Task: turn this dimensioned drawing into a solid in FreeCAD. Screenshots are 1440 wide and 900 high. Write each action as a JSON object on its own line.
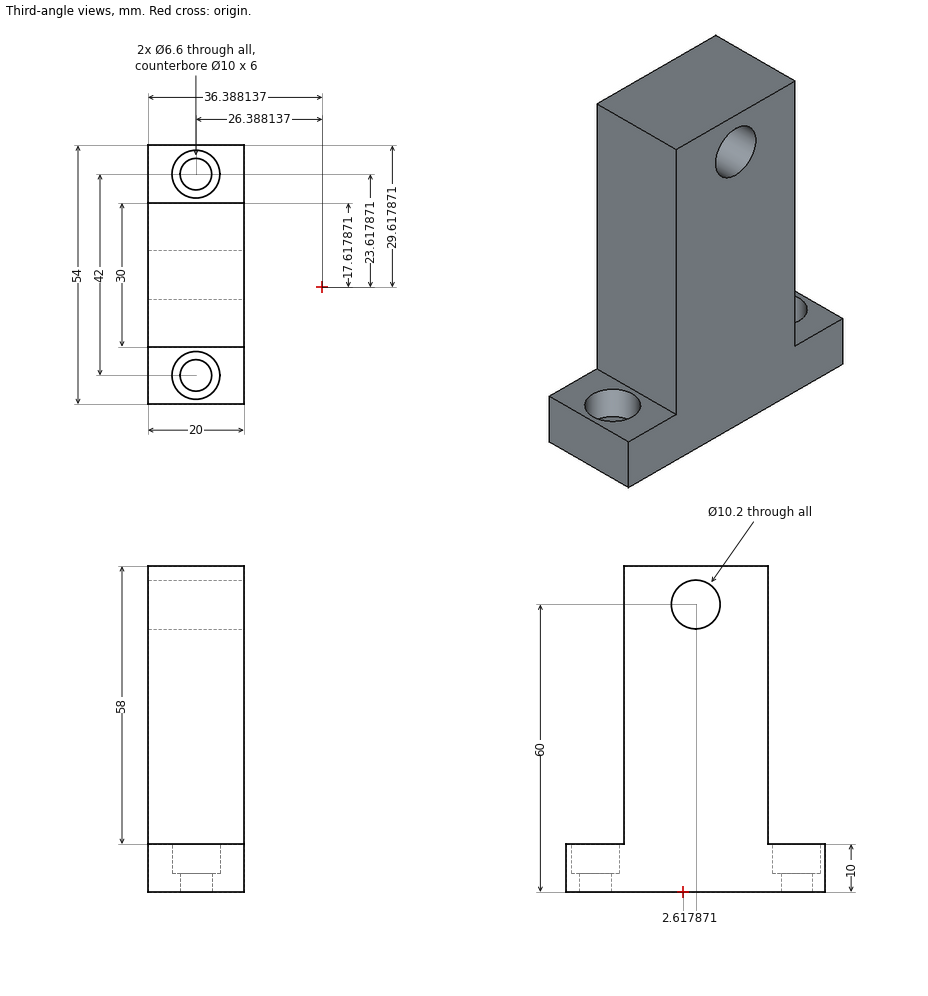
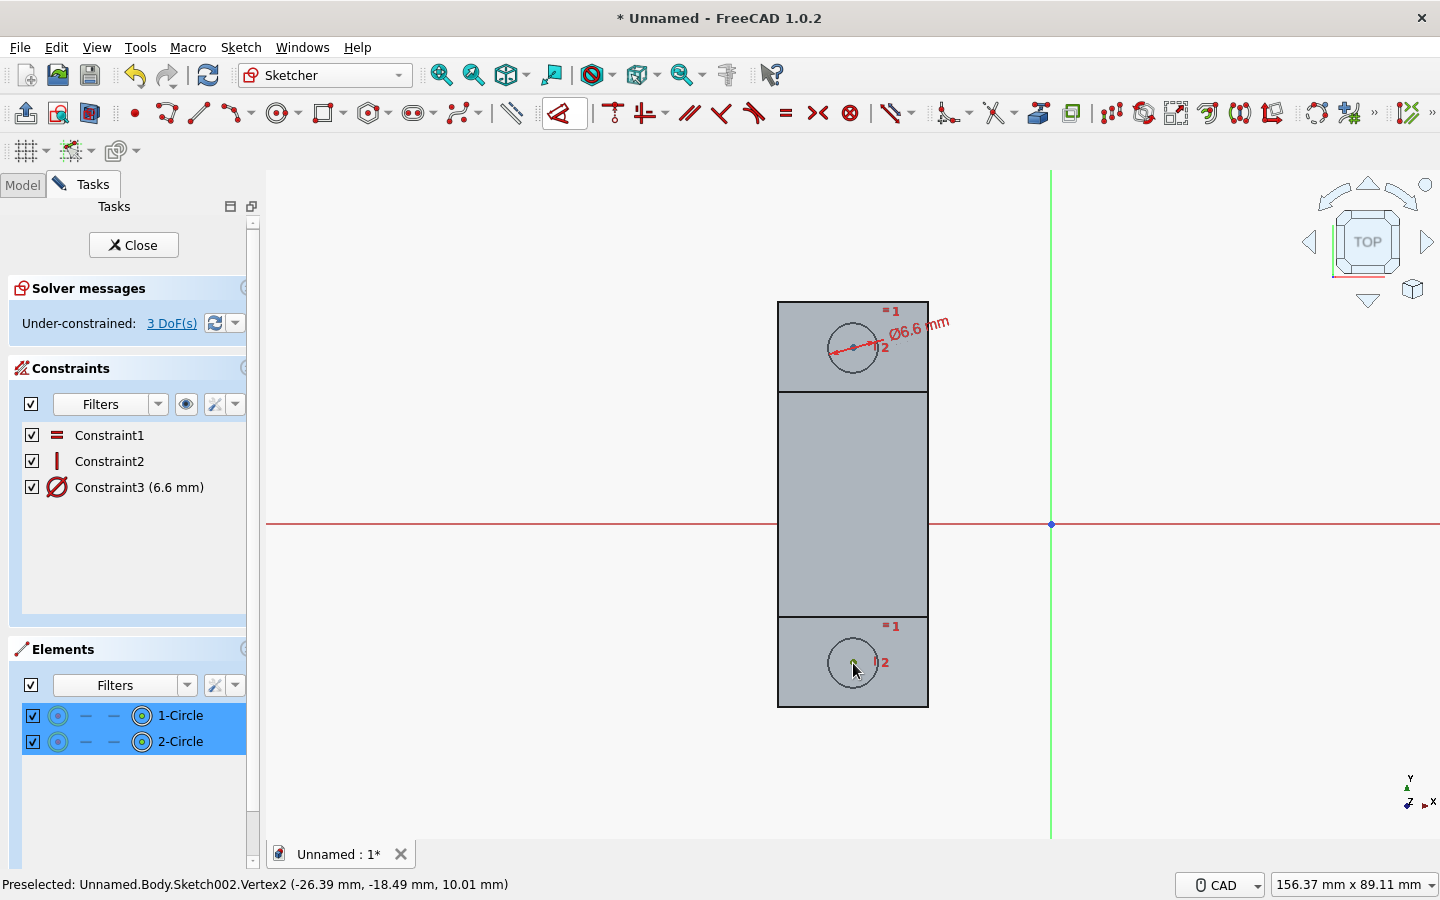
{"action": "key", "text": "i"}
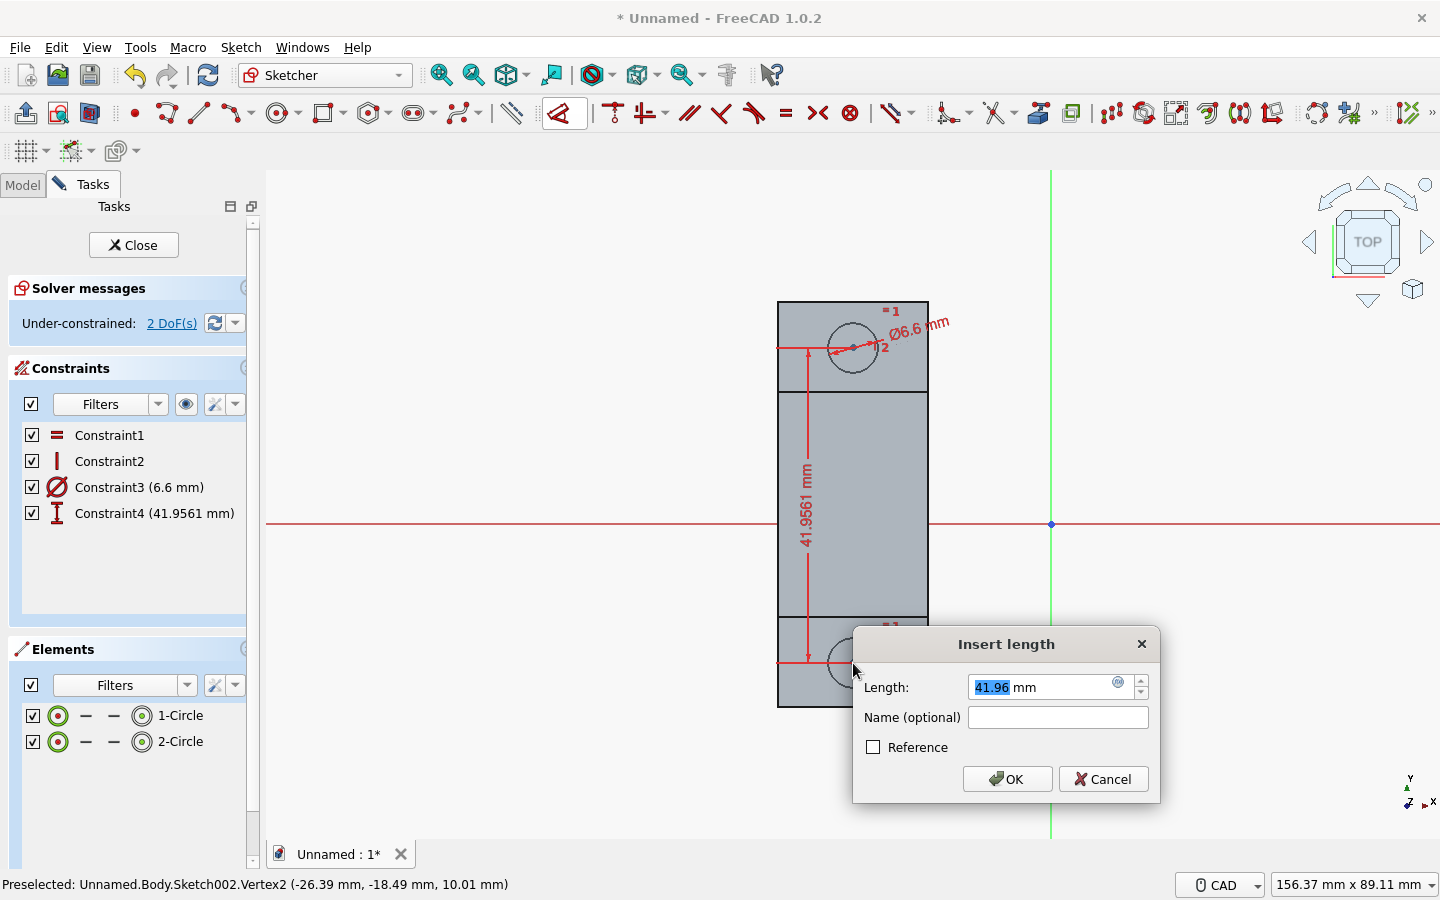
{"action": "type", "text": "42"}
{"action": "key", "text": "Return"}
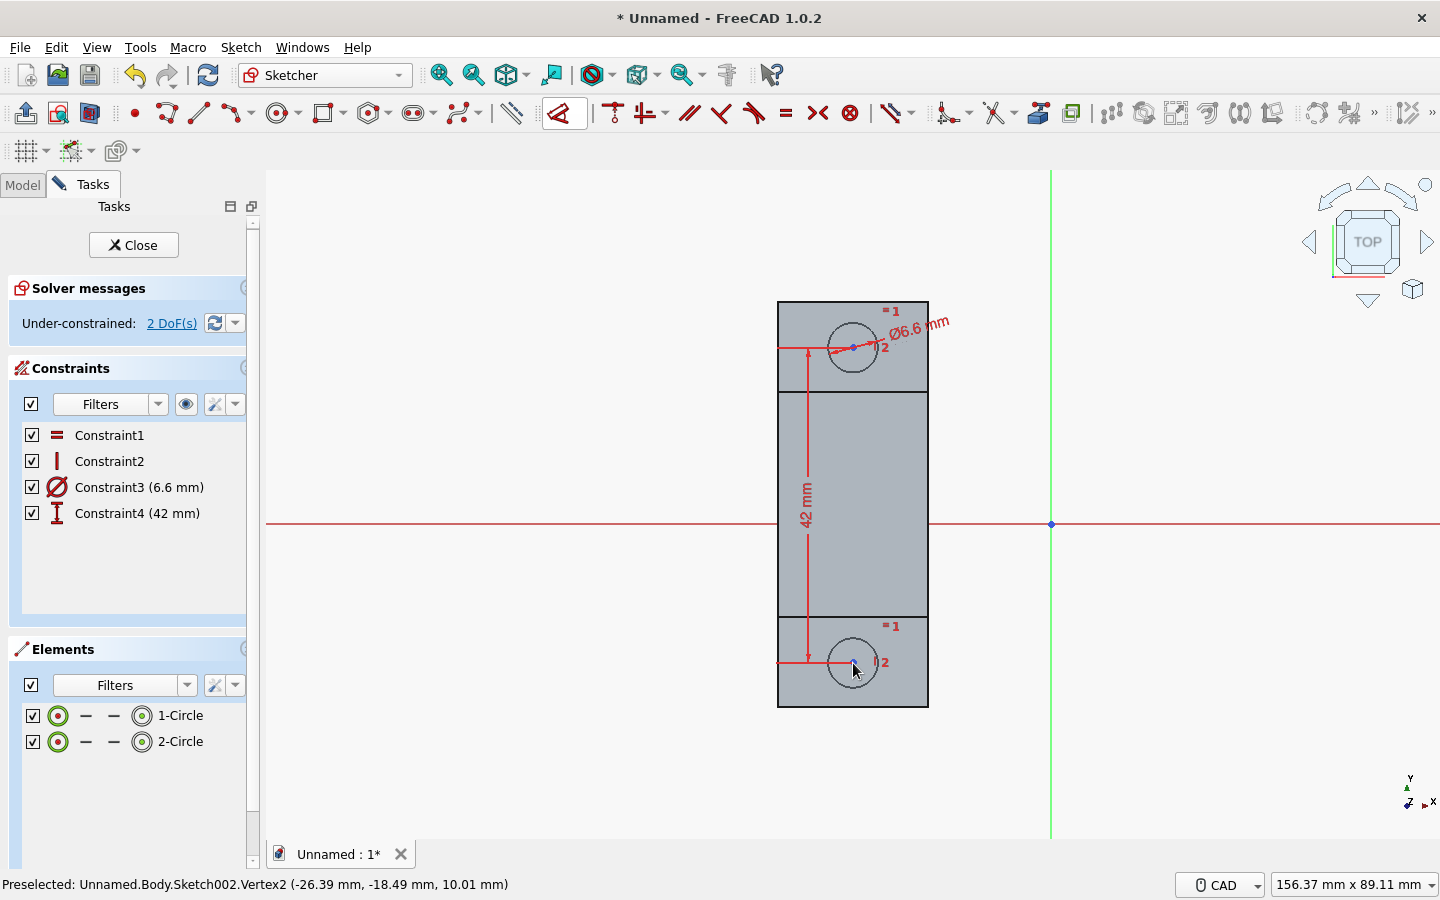
{"action": "left_click", "coordinate": [853, 348]}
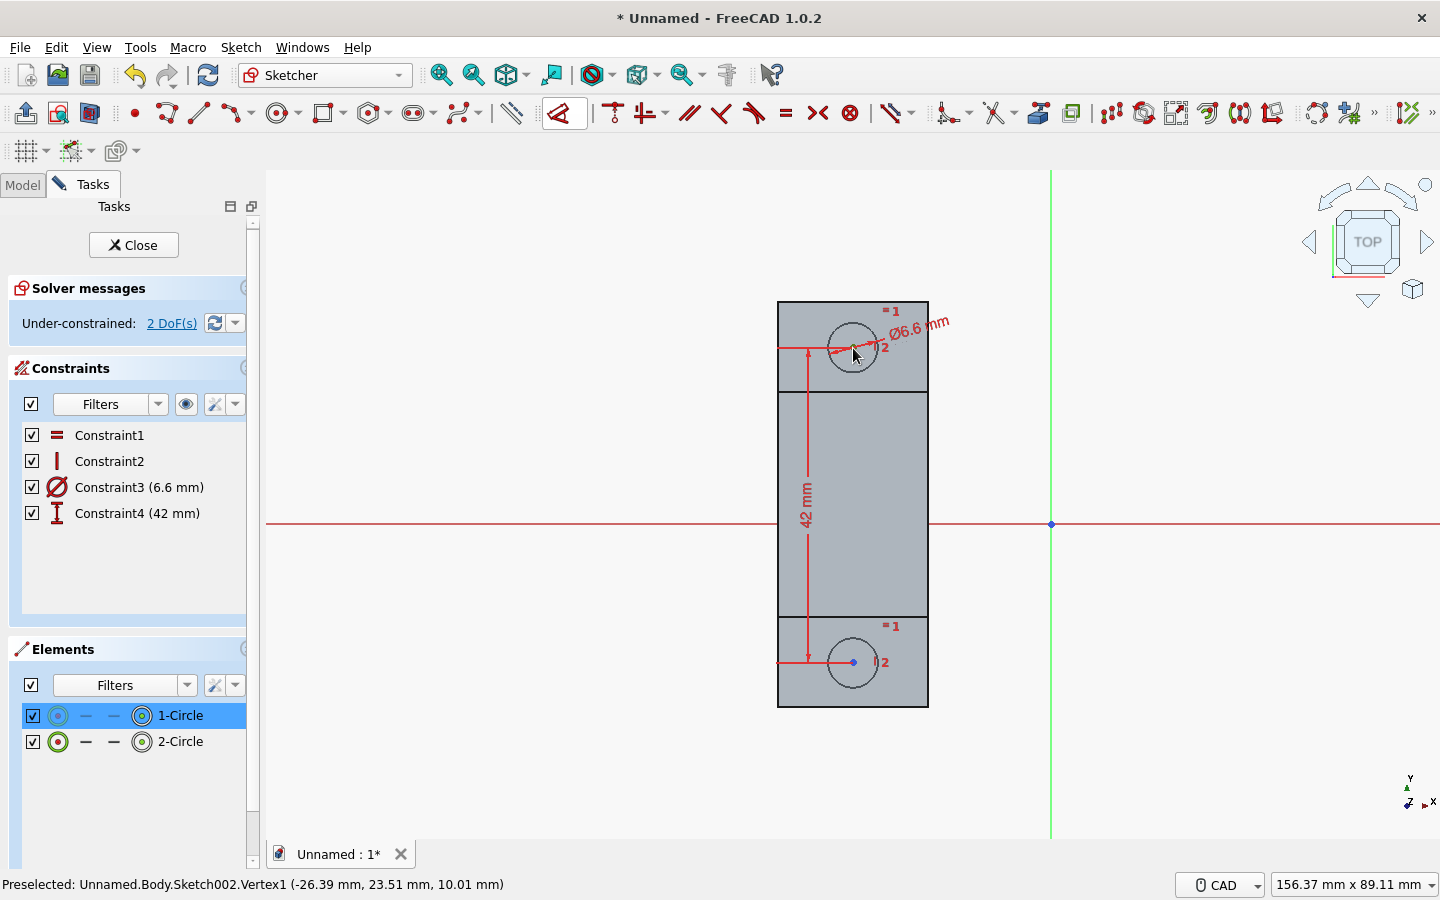
{"action": "key", "text": "l"}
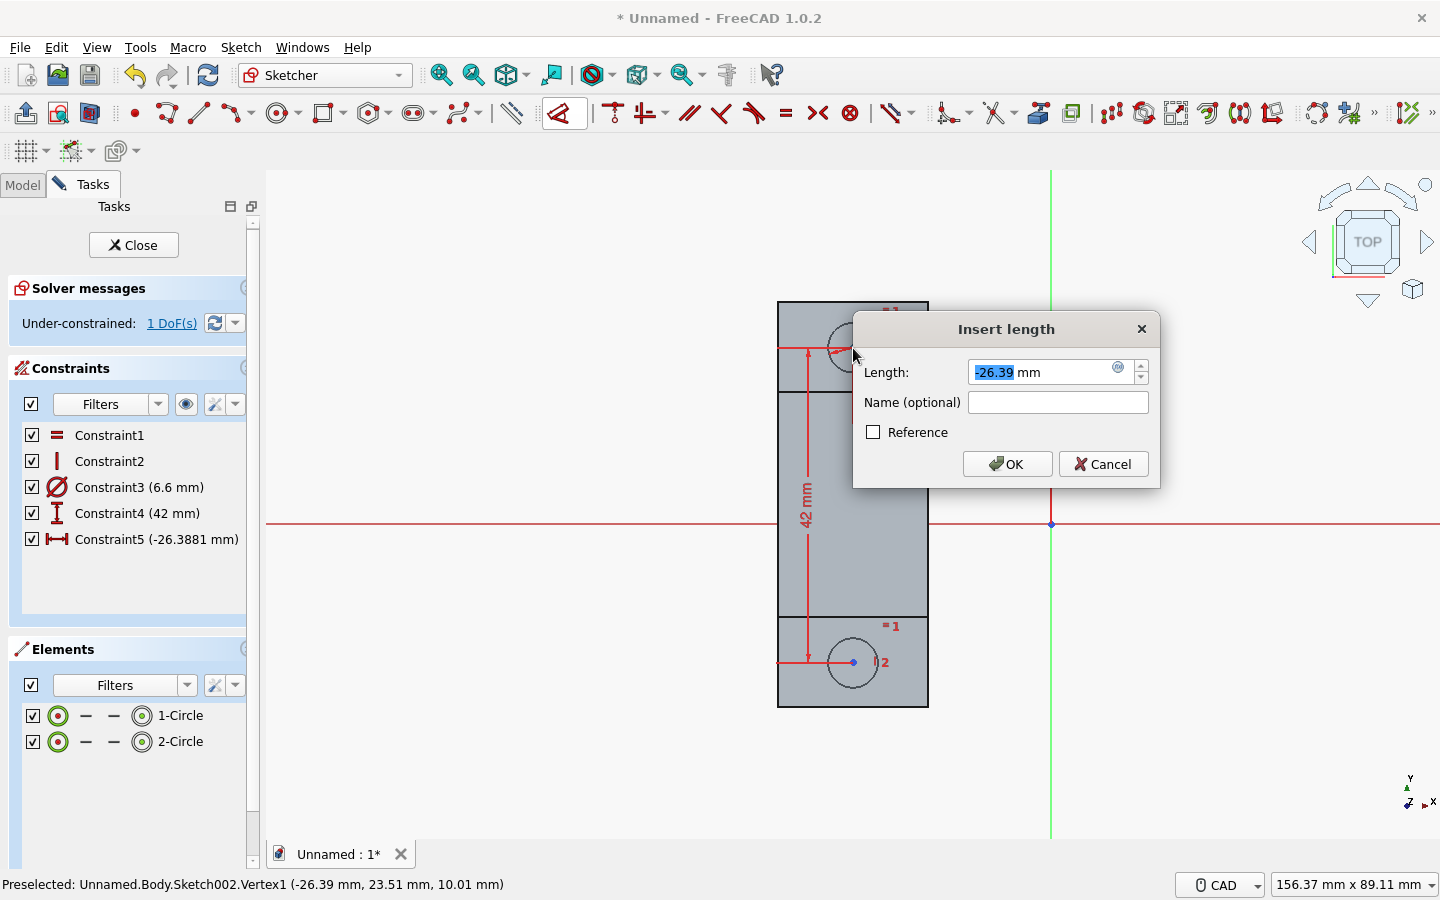
{"action": "type", "text": "-26.388137"}
{"action": "key", "text": "Return"}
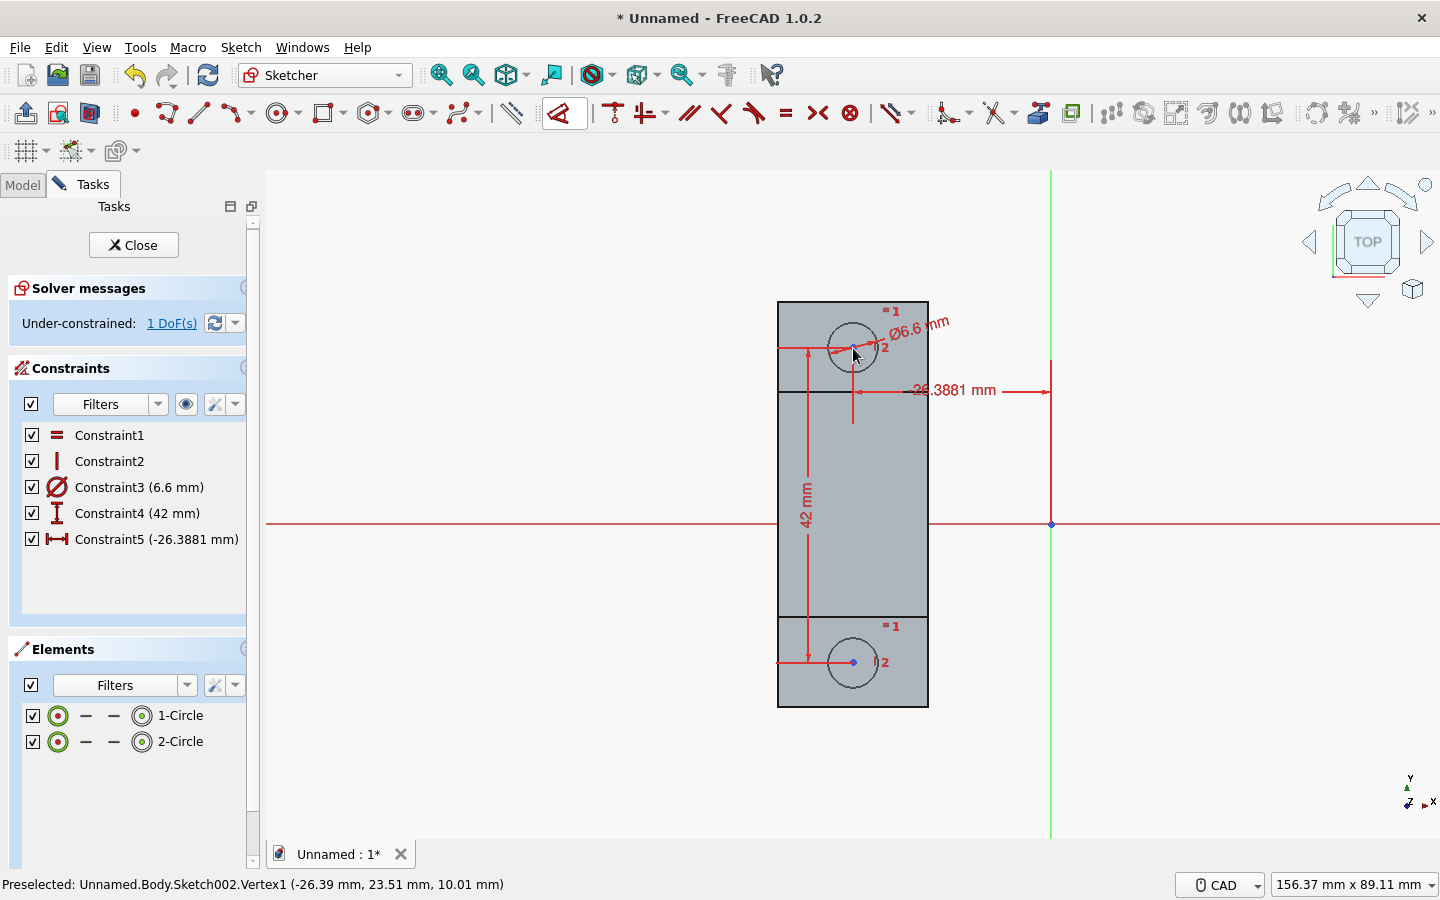
{"action": "left_click", "coordinate": [853, 348]}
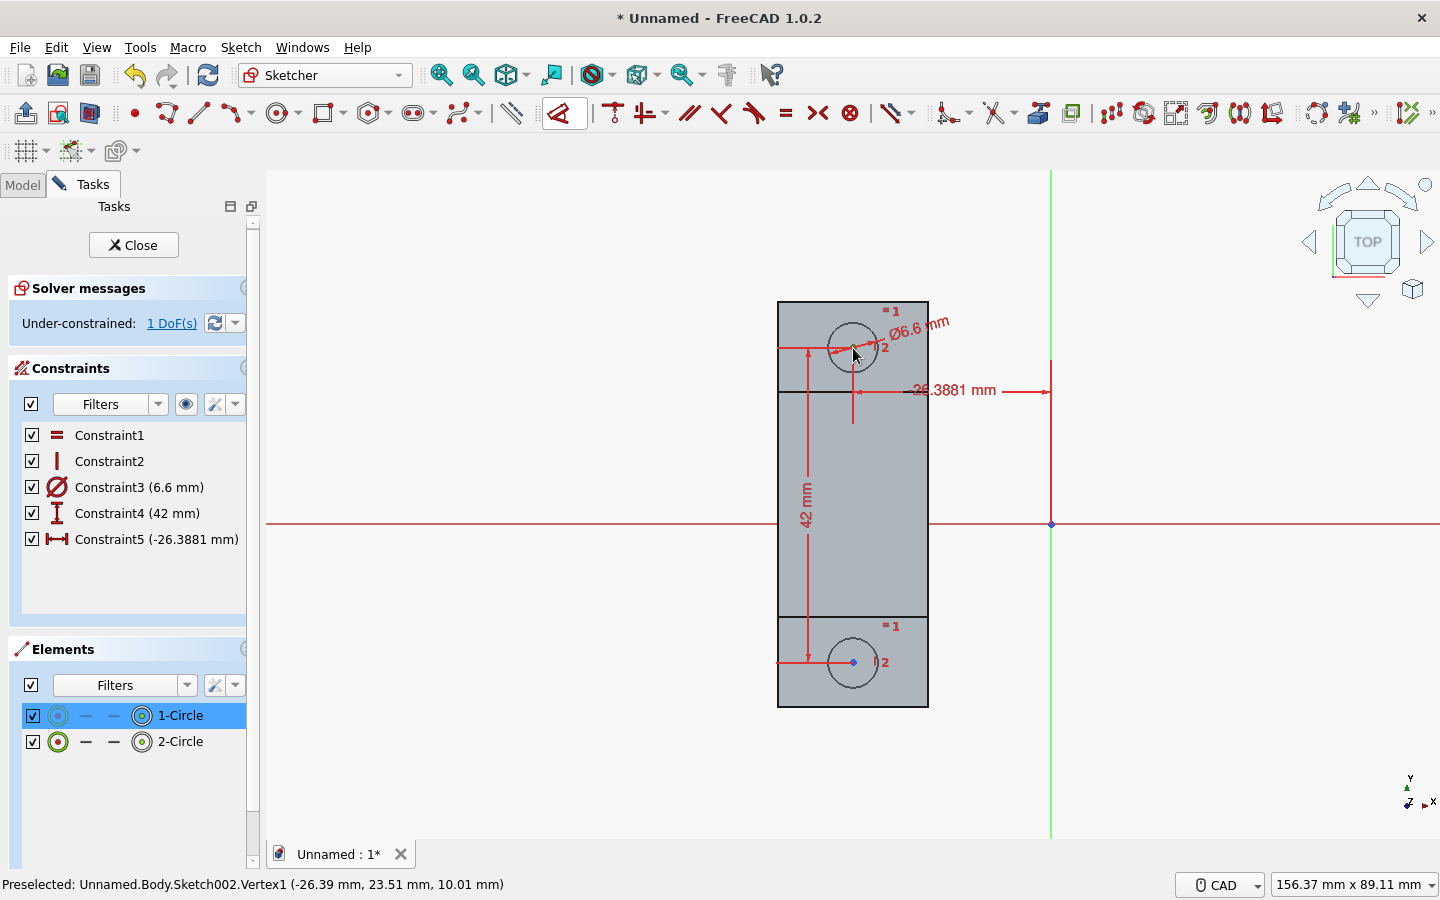
{"action": "left_click", "coordinate": [582, 114]}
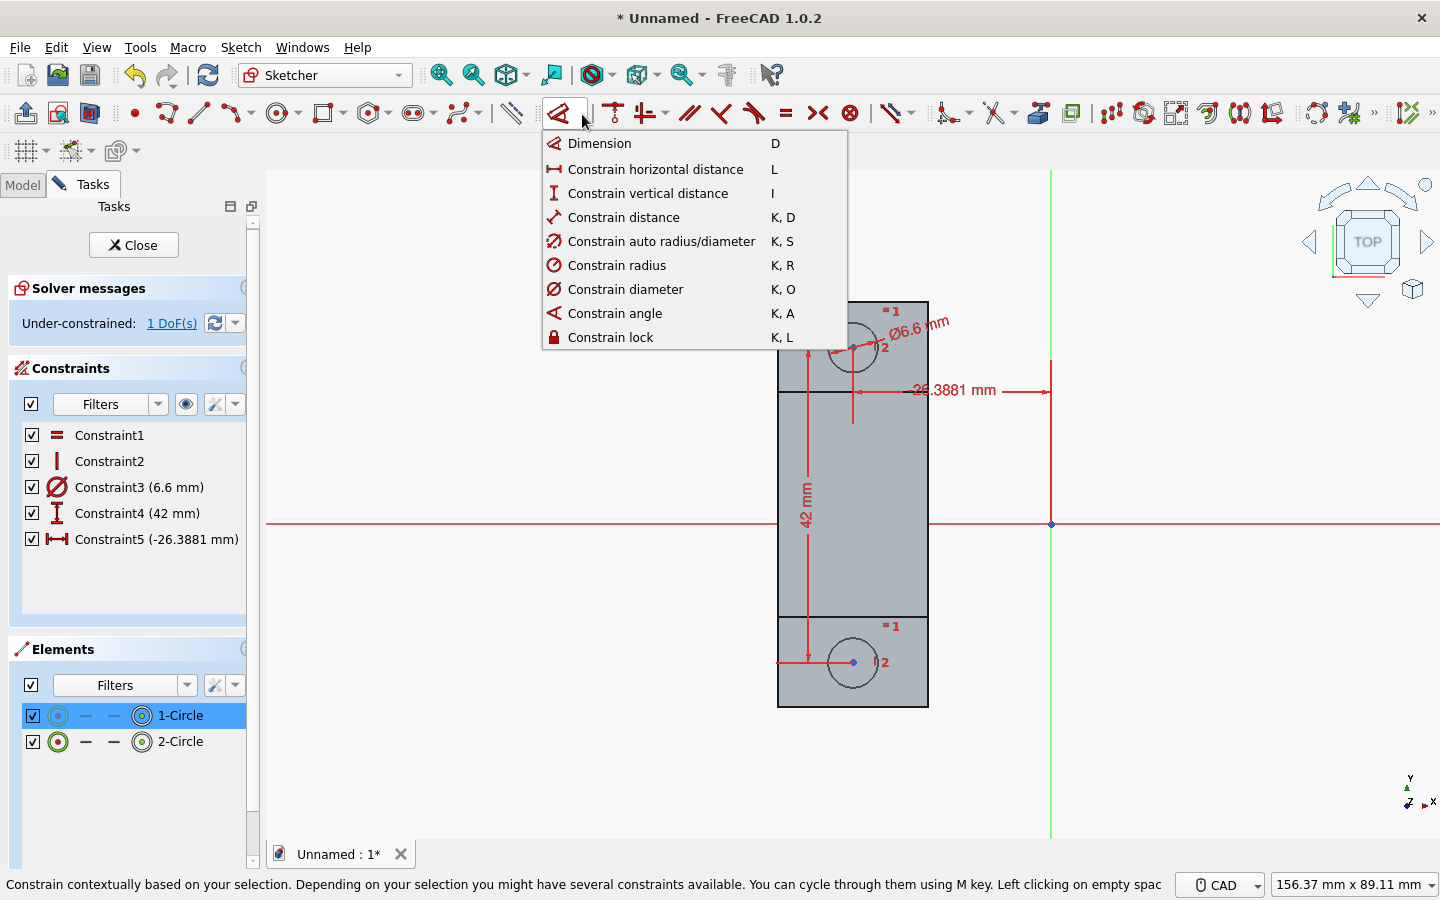
{"action": "left_click", "coordinate": [695, 193]}